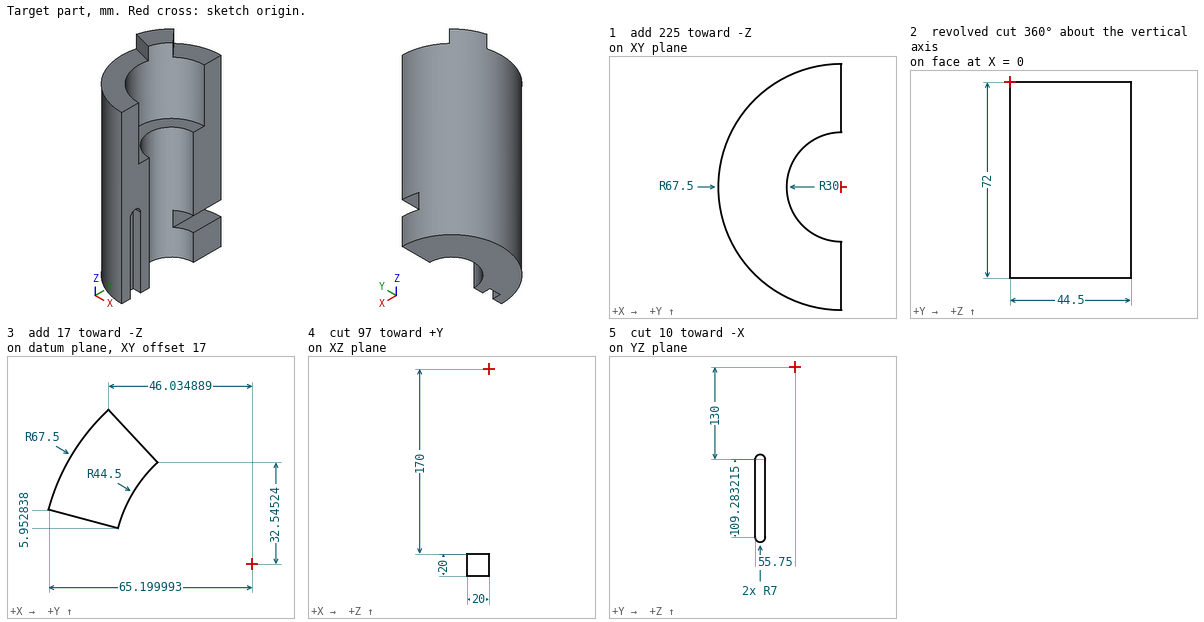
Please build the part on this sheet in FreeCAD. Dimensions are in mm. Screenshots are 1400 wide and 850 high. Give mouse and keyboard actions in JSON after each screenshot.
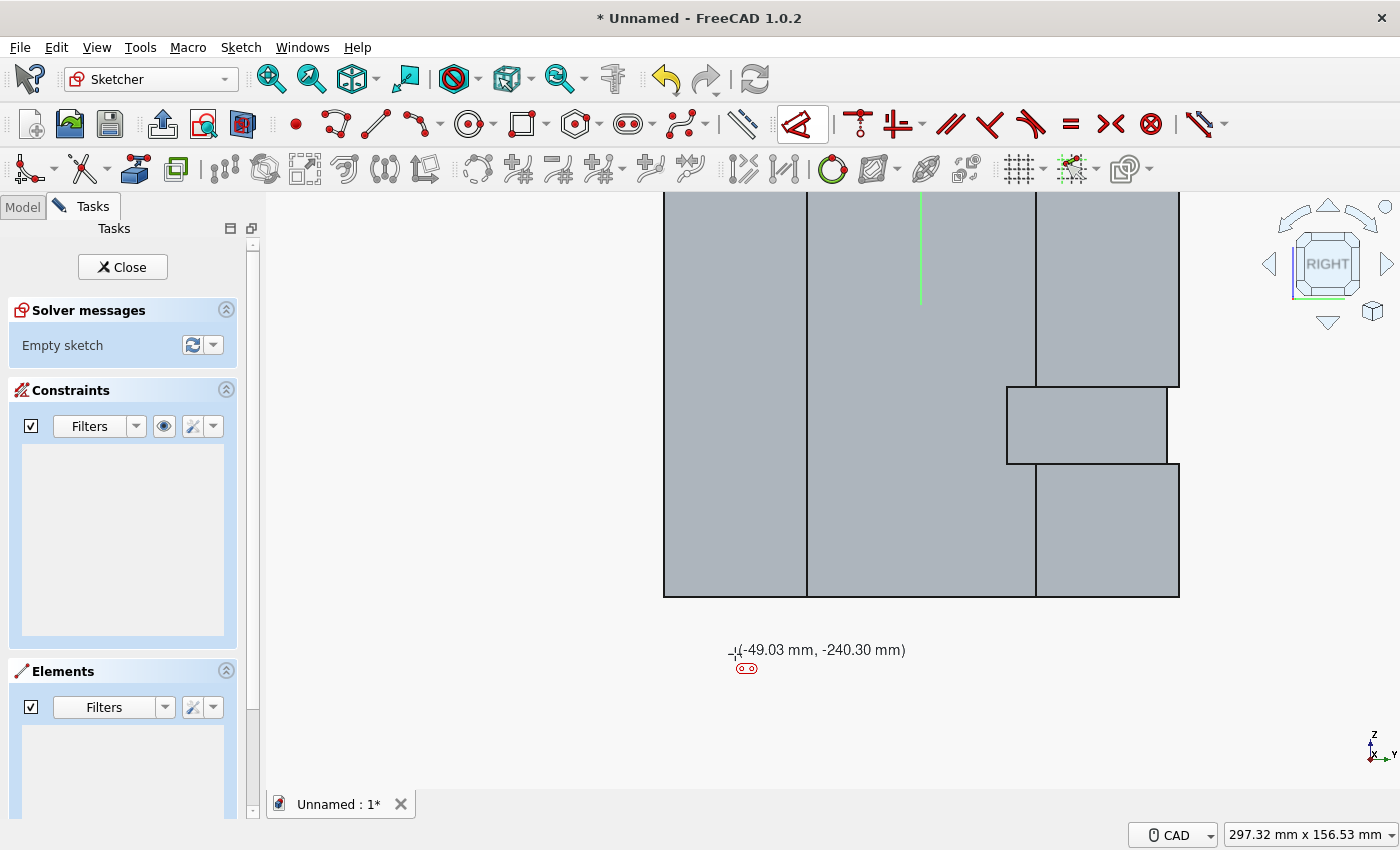
{"action": "left_click", "coordinate": [735, 651]}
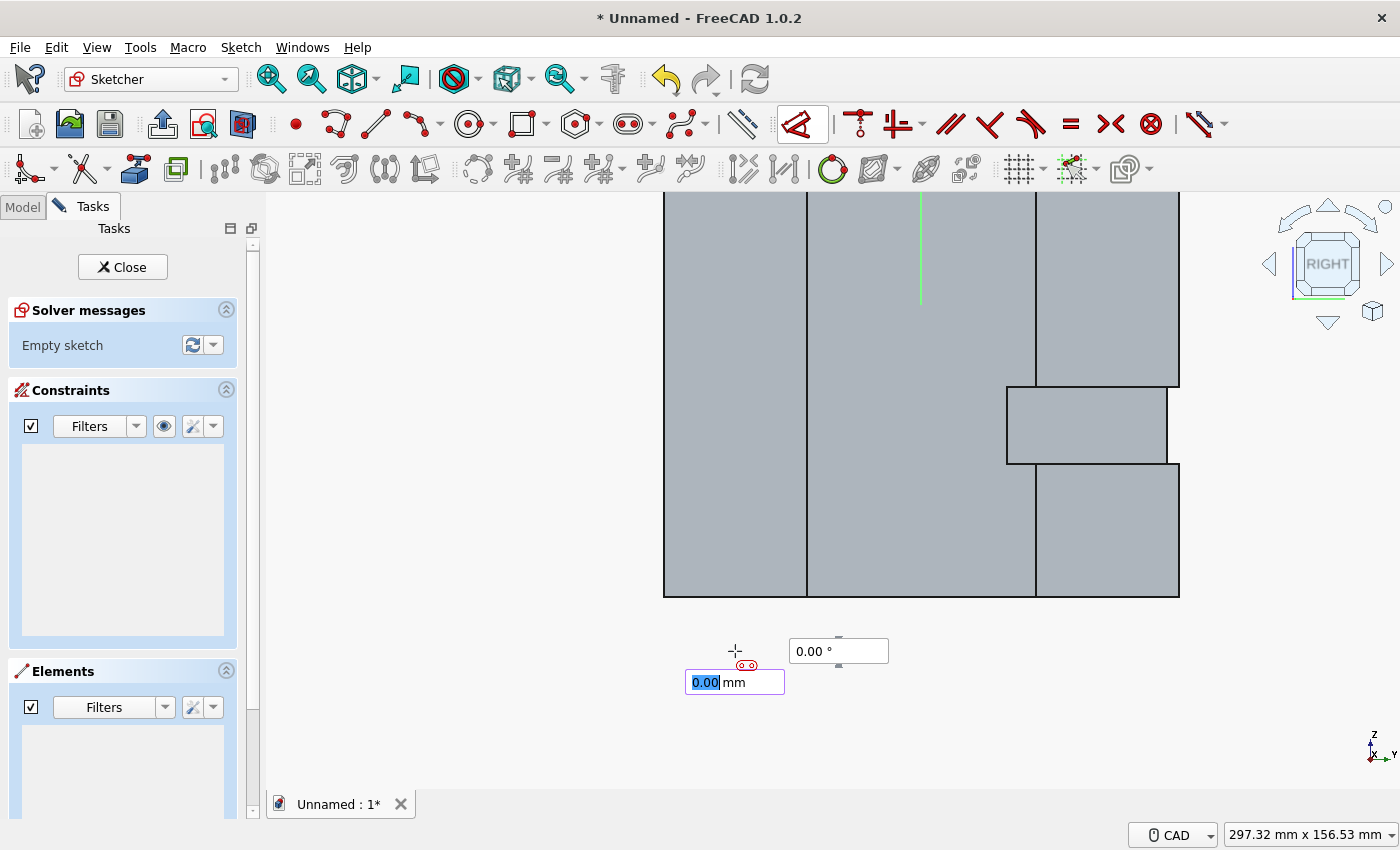
{"action": "left_click", "coordinate": [735, 235]}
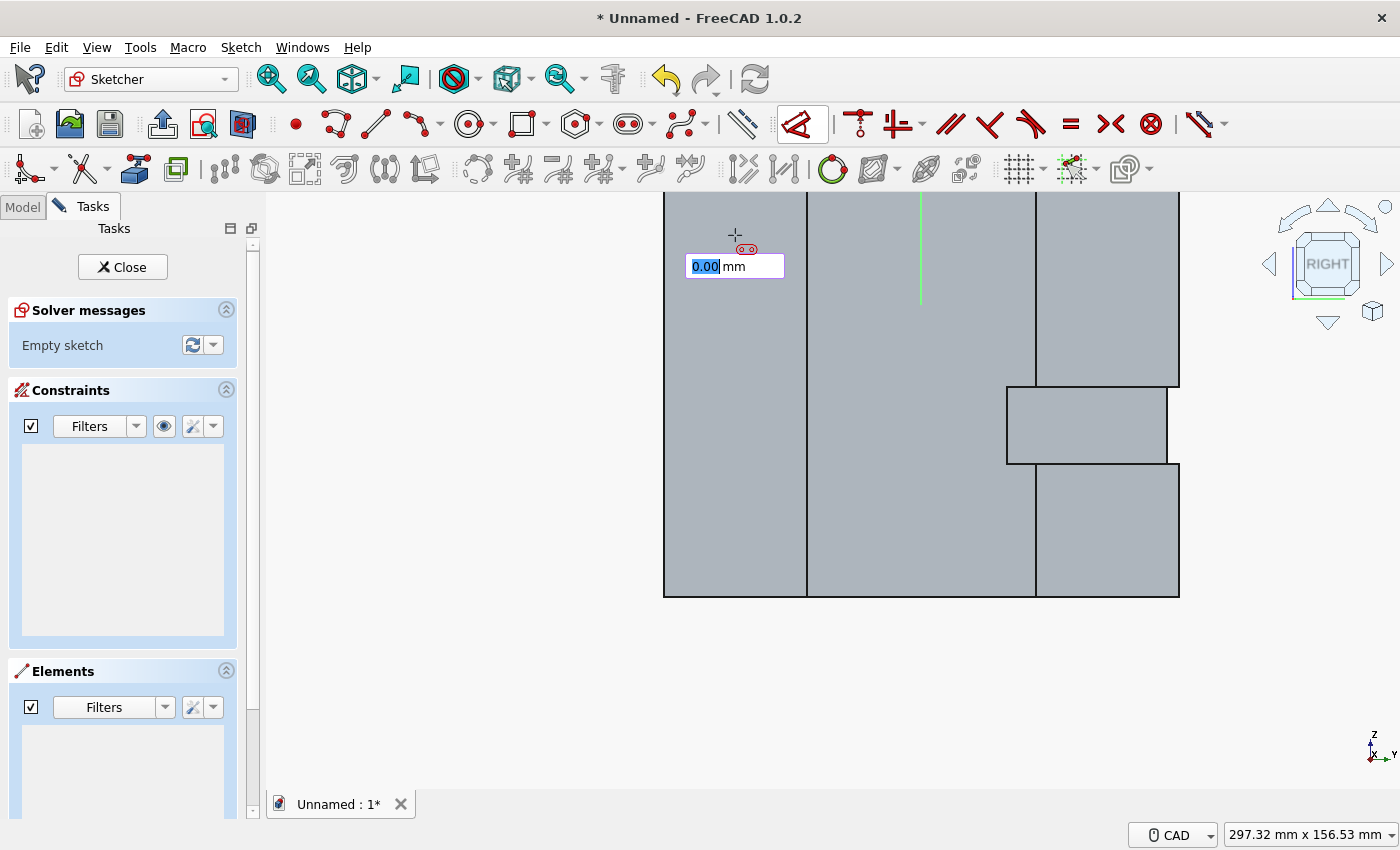
{"action": "left_click", "coordinate": [709, 443]}
{"action": "key", "text": "Escape"}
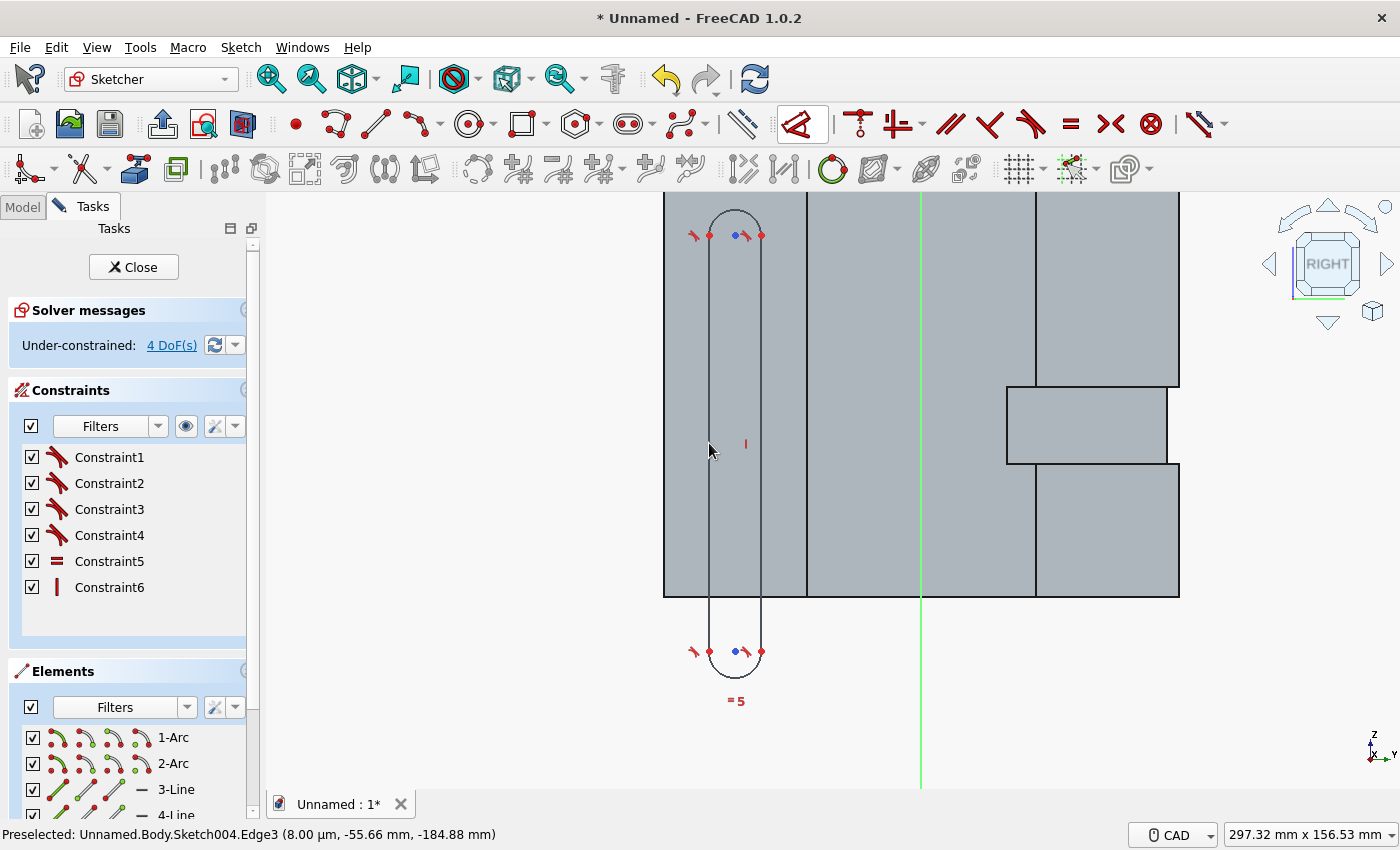
{"action": "scroll", "coordinate": [720, 673], "scroll_direction": "up", "scroll_amount": 2}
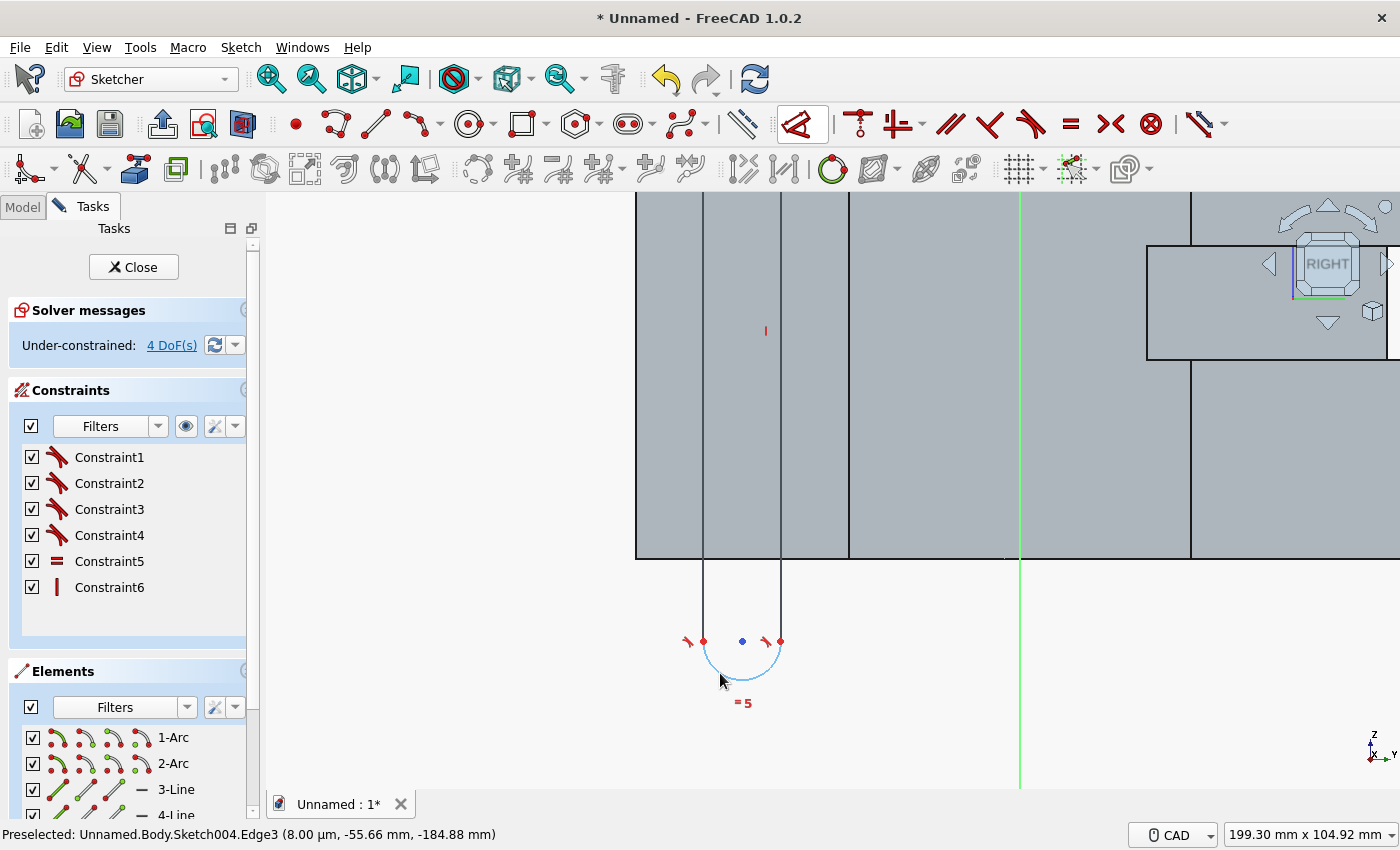
{"action": "left_click", "coordinate": [719, 673]}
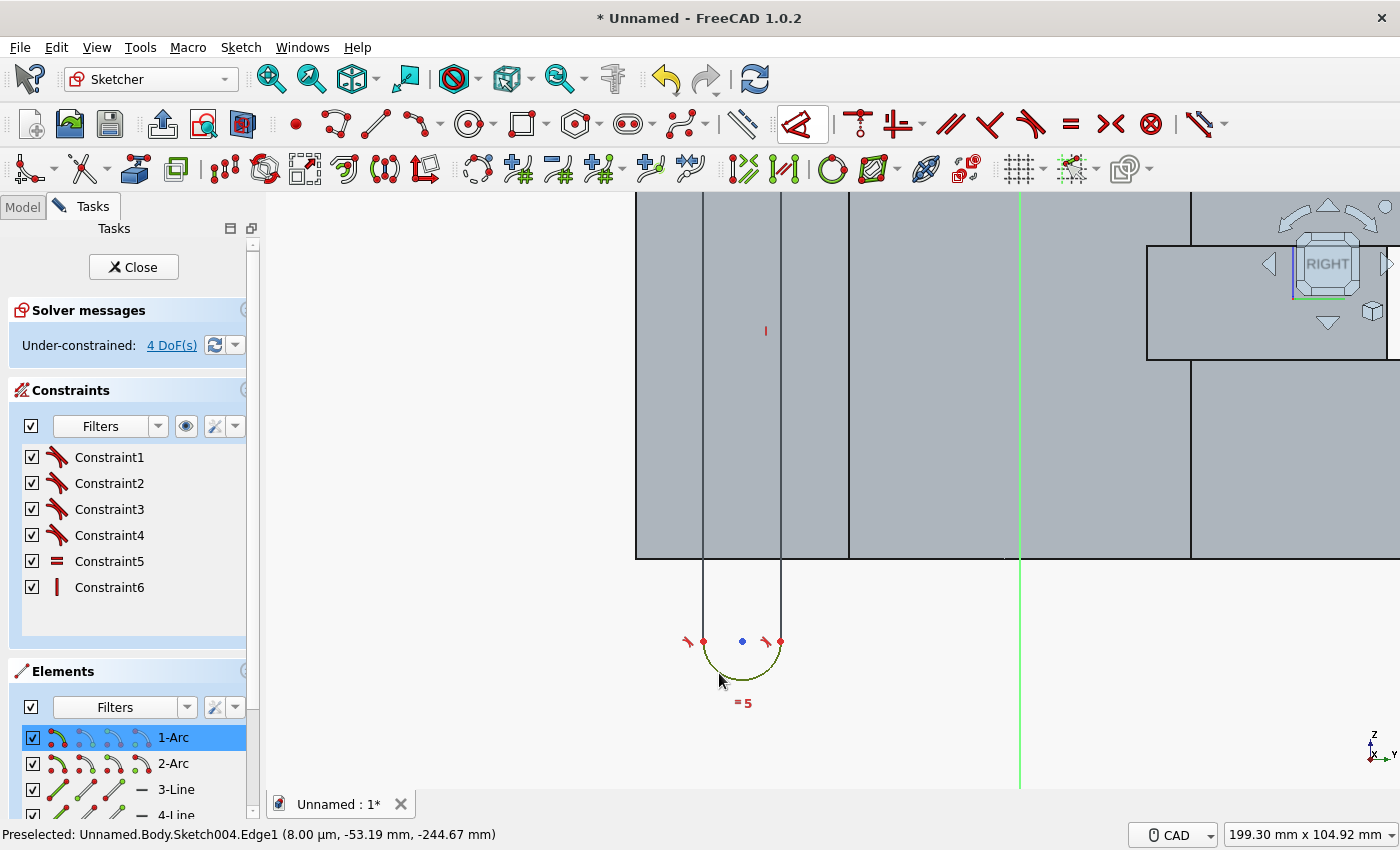
{"action": "key", "text": "k r"}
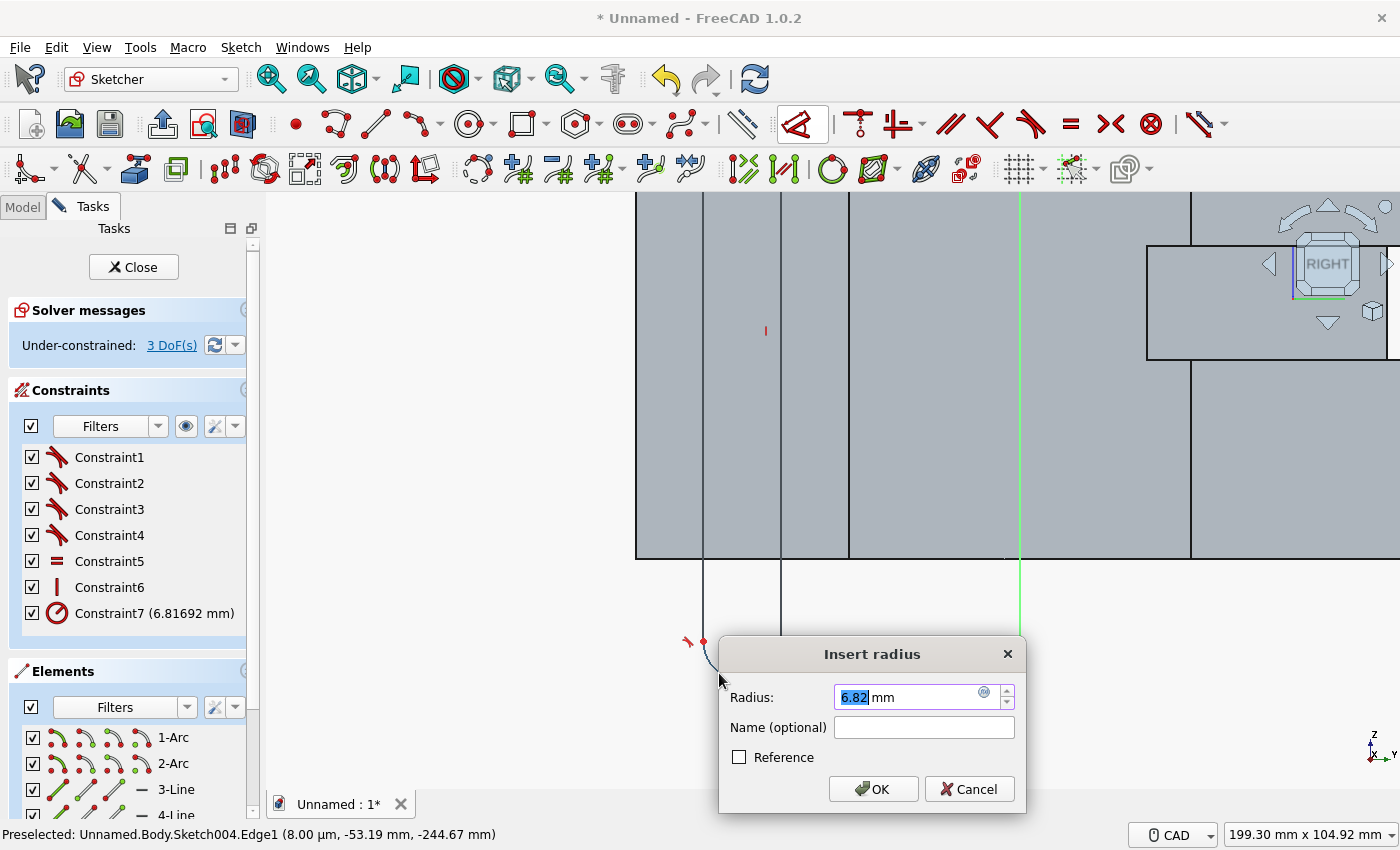
{"action": "type", "text": "7"}
{"action": "key", "text": "Return"}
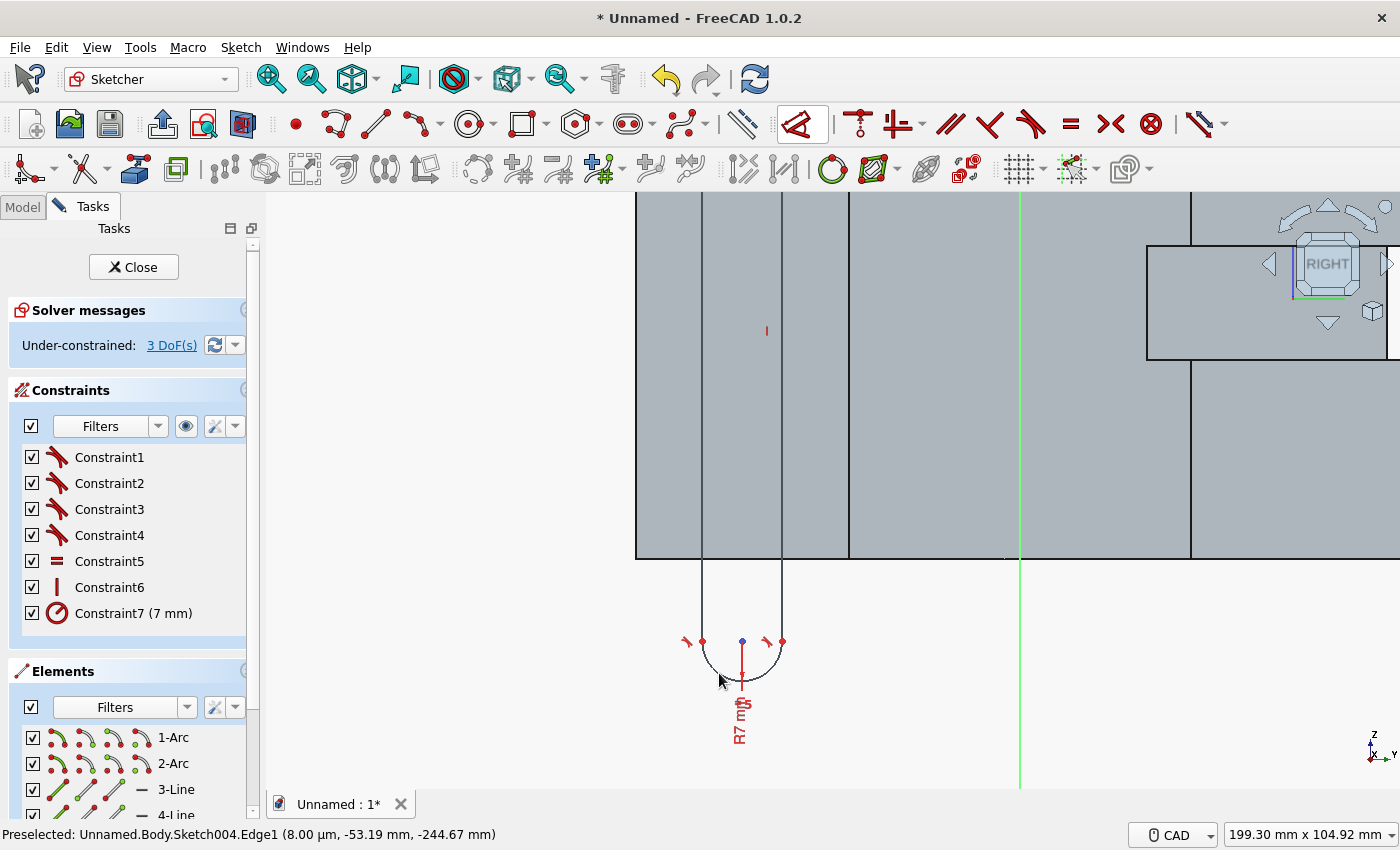
{"action": "scroll", "coordinate": [733, 658], "scroll_direction": "down", "scroll_amount": 7}